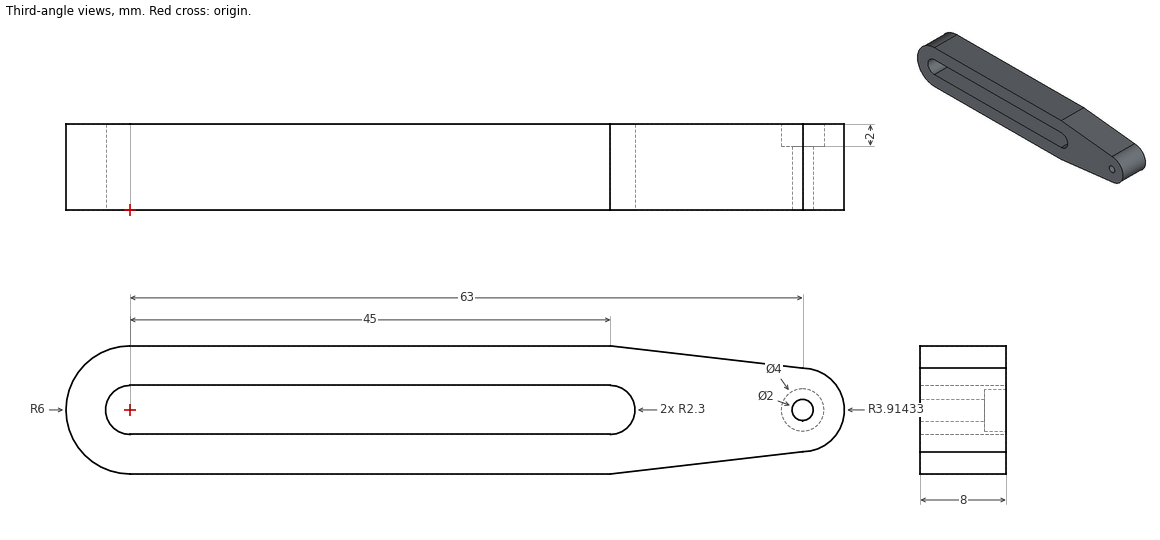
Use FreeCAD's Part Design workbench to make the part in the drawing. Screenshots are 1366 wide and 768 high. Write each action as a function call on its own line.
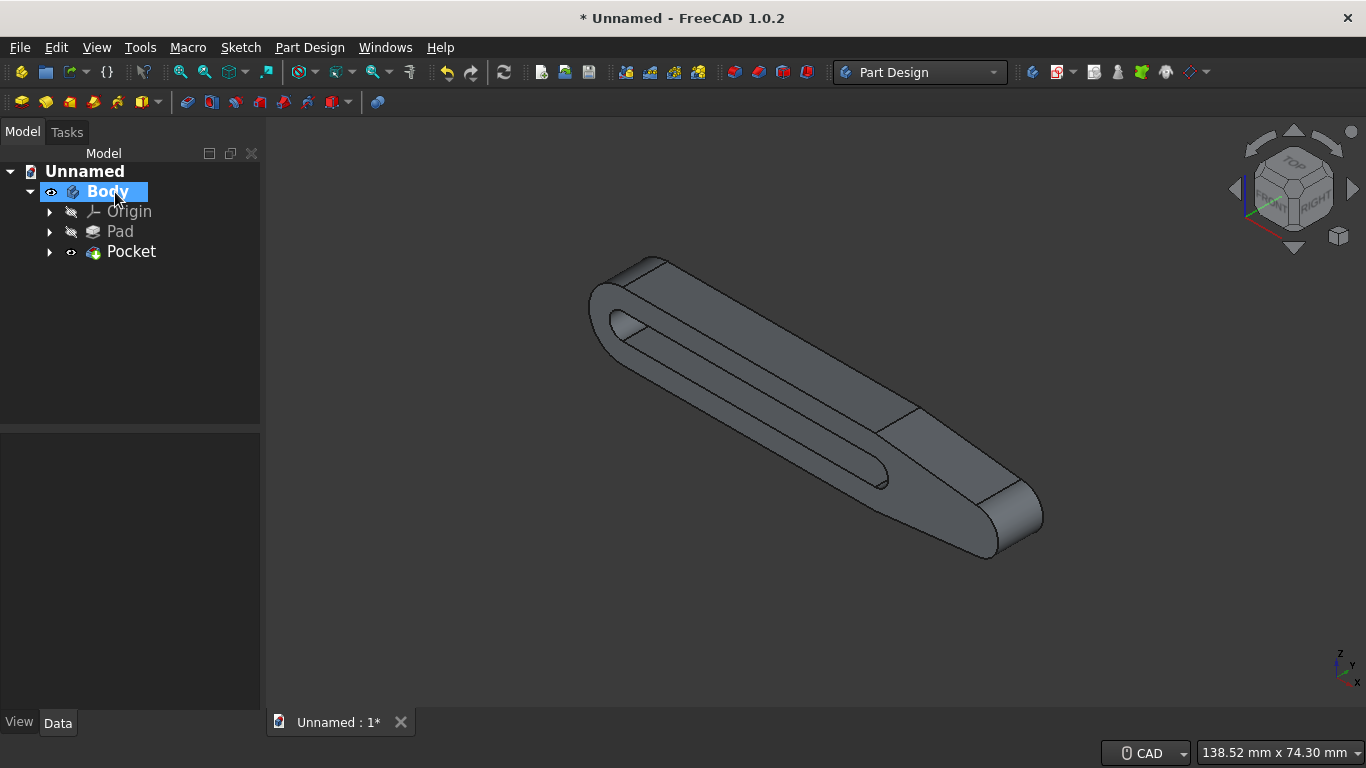
click(969, 525)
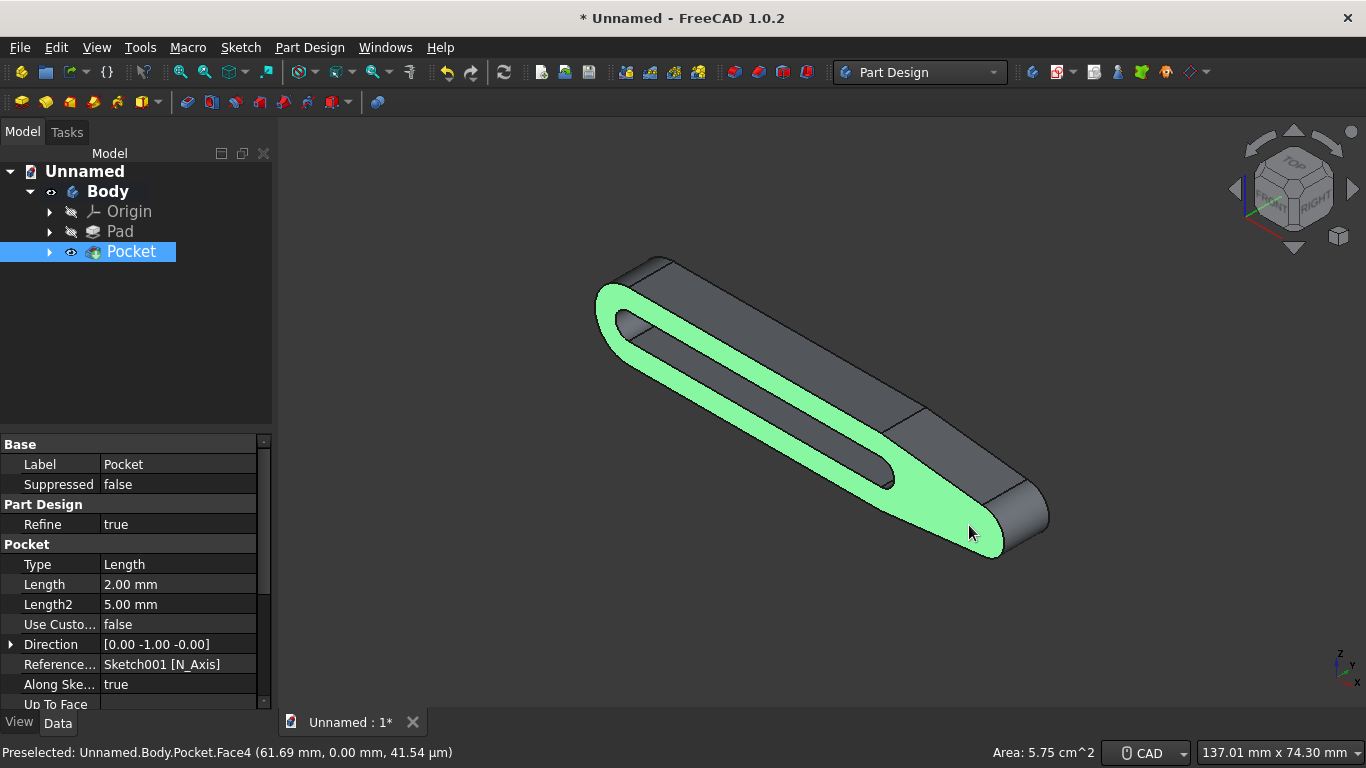
click(1058, 72)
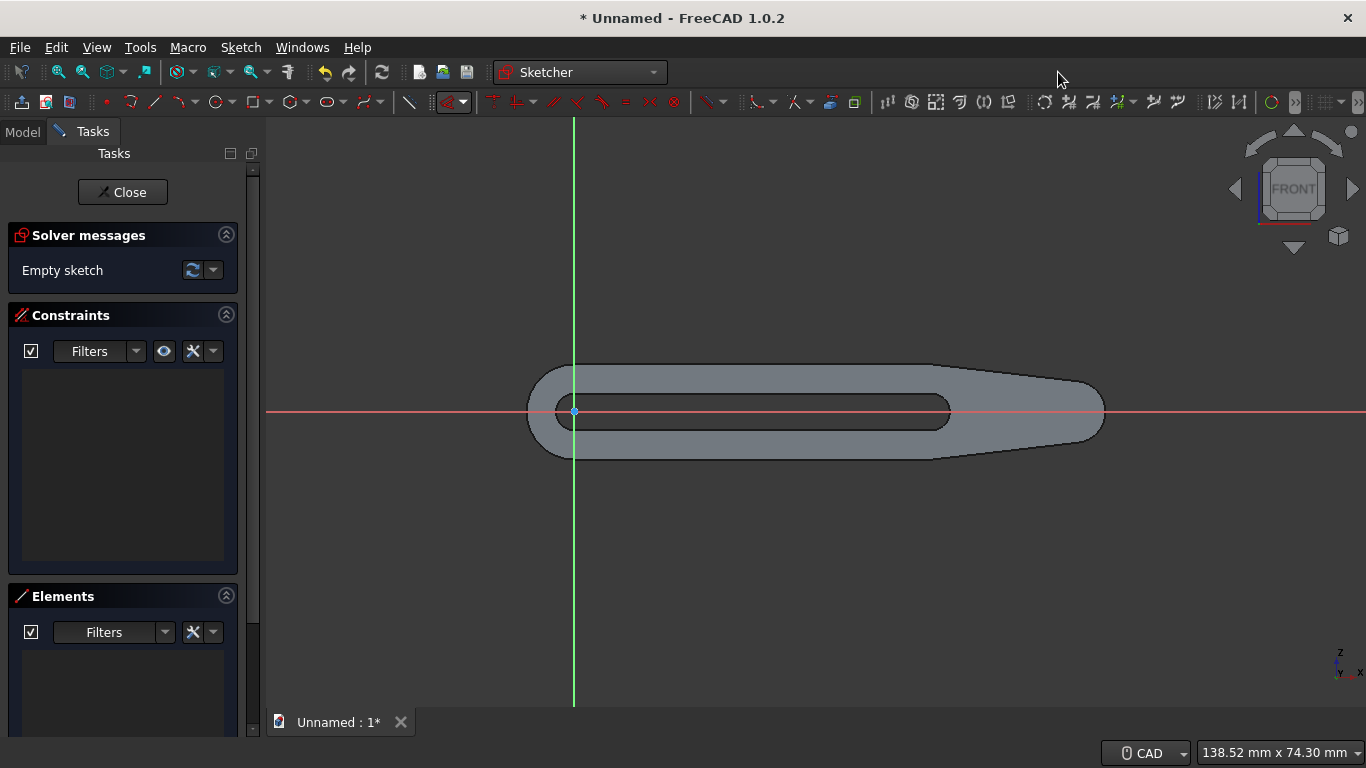
scroll(1092, 412, up, 15)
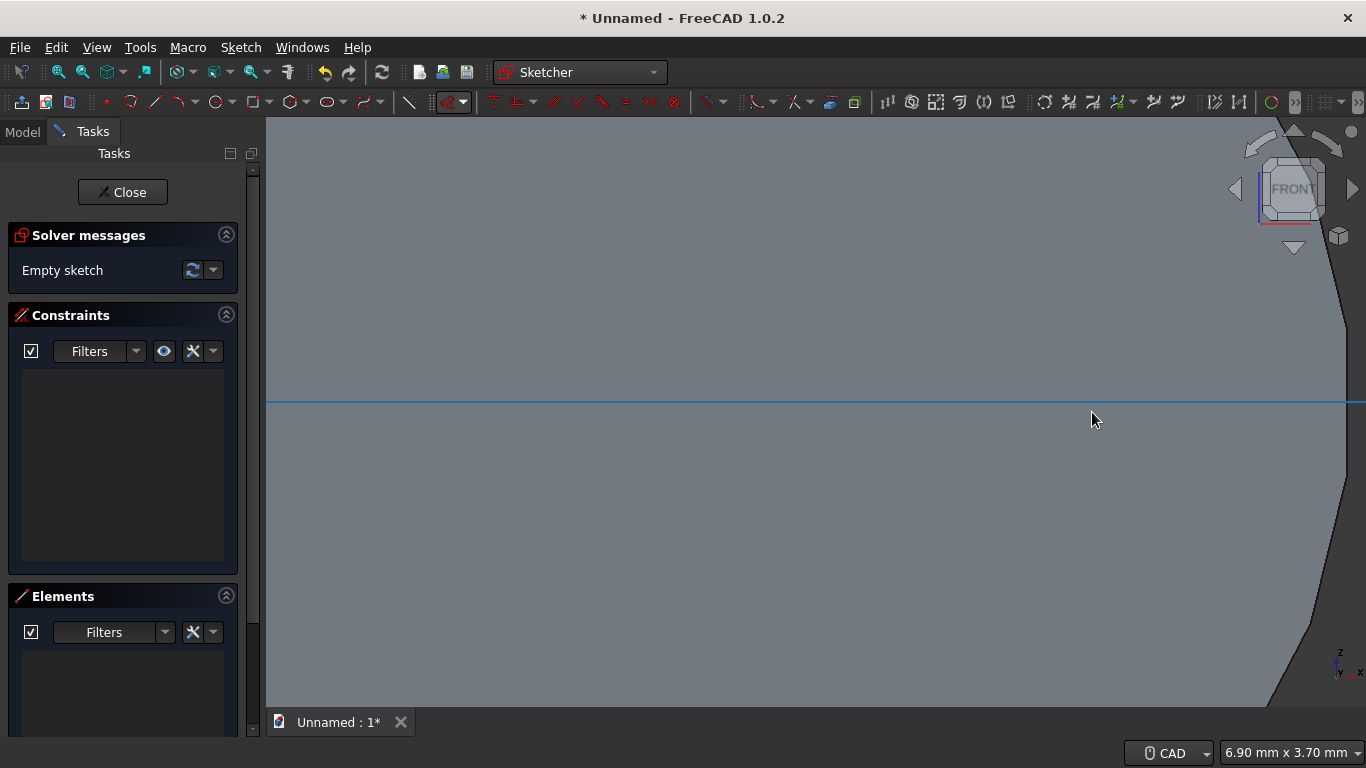
click(216, 102)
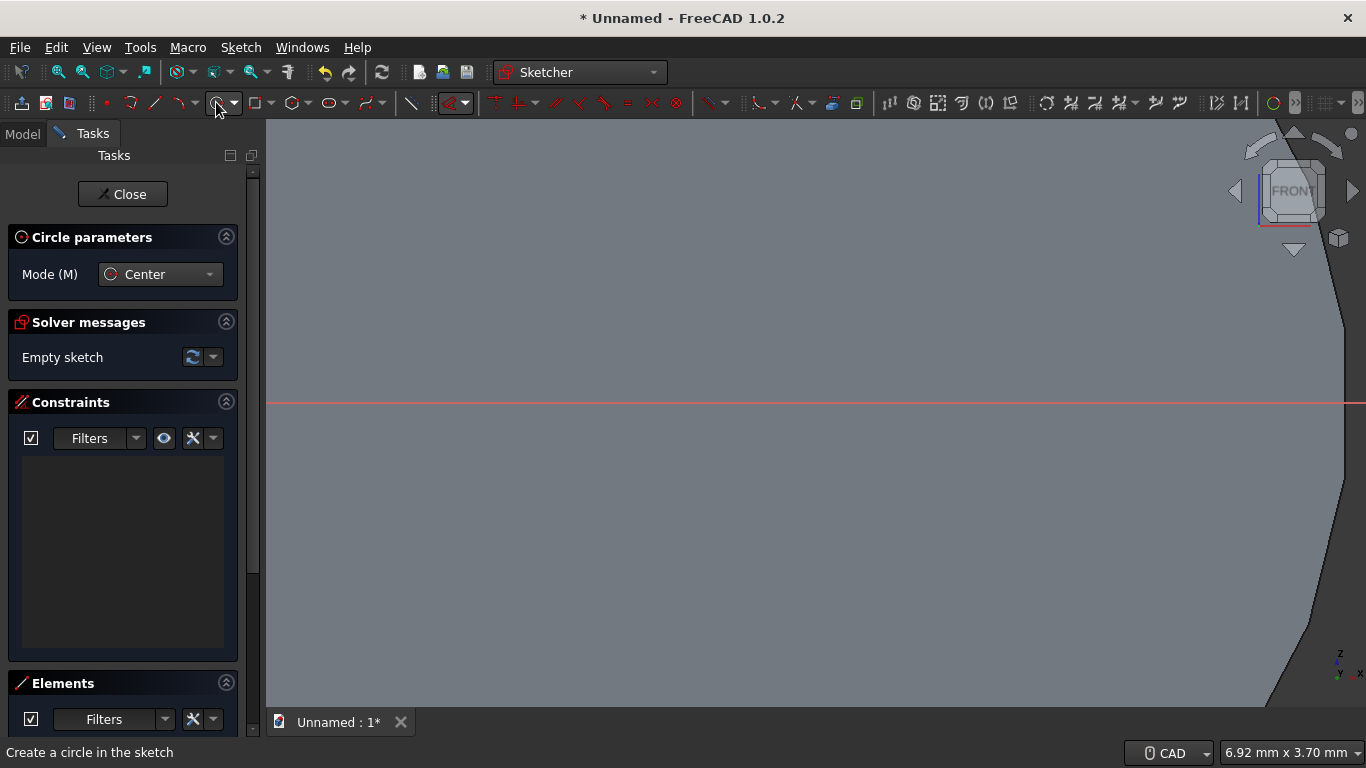
click(727, 403)
move(840, 291)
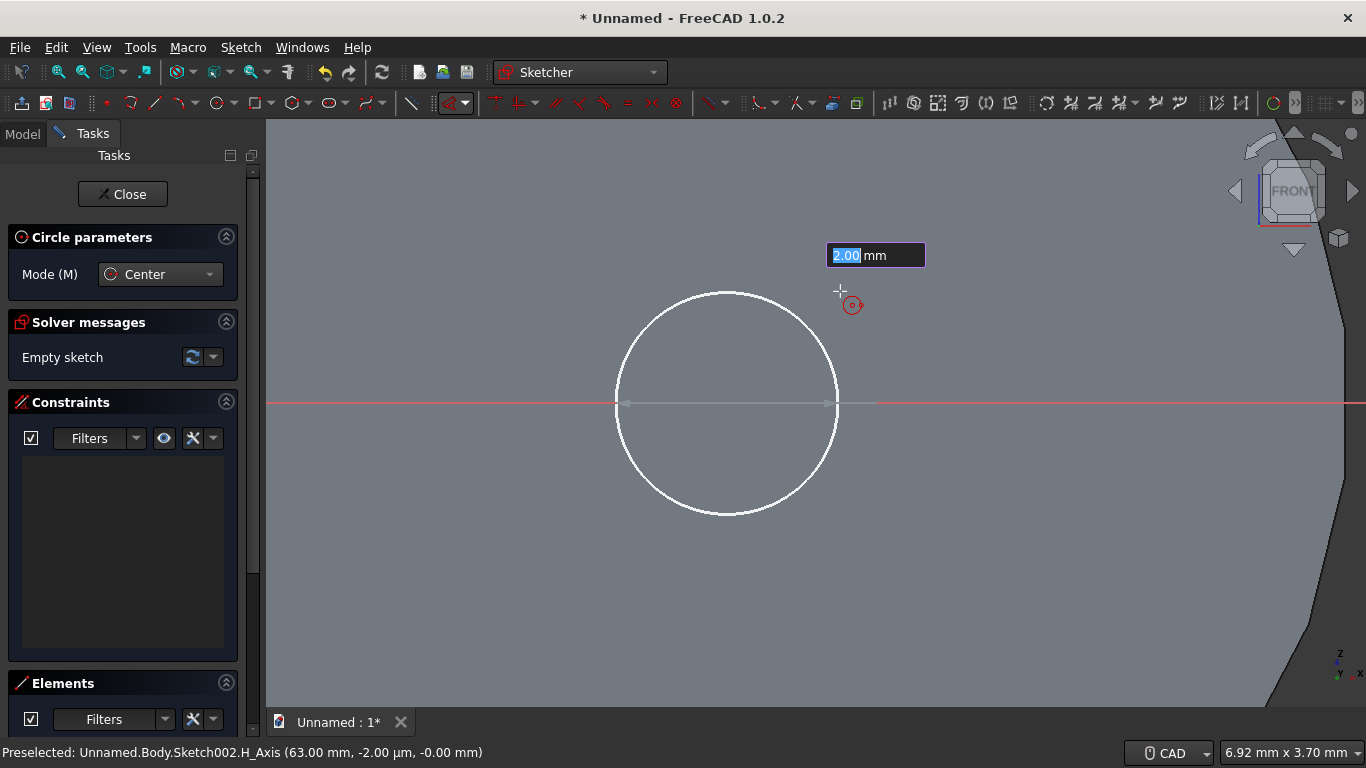
text(2)
key(Return)
key(Escape)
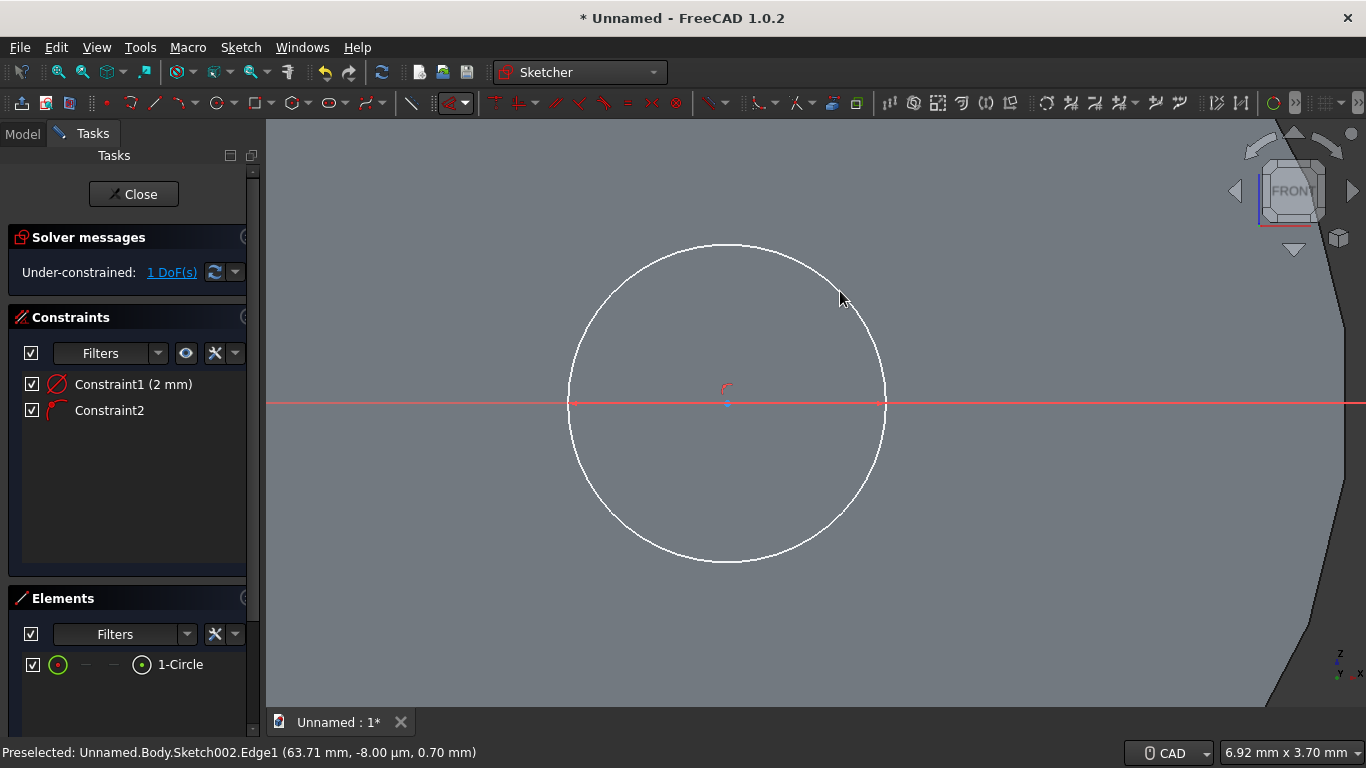
click(727, 403)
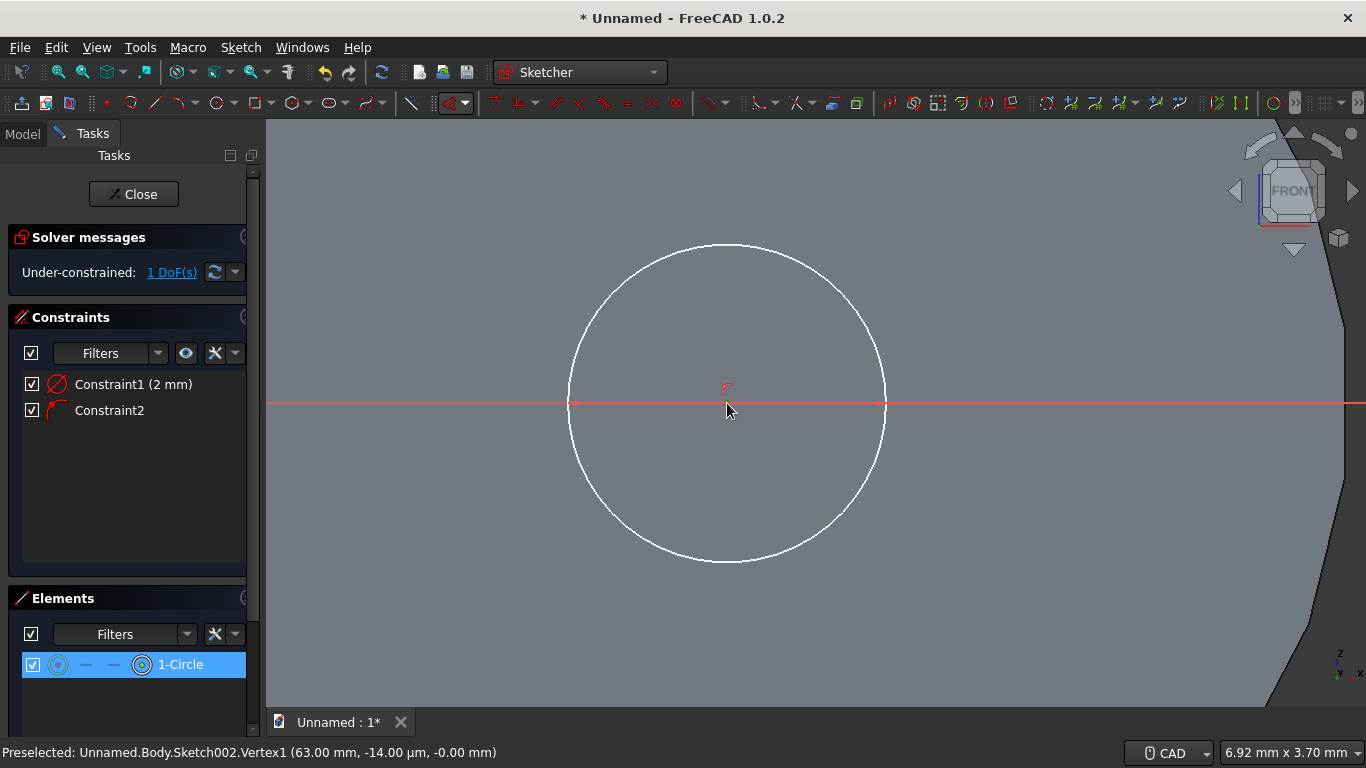
key(l)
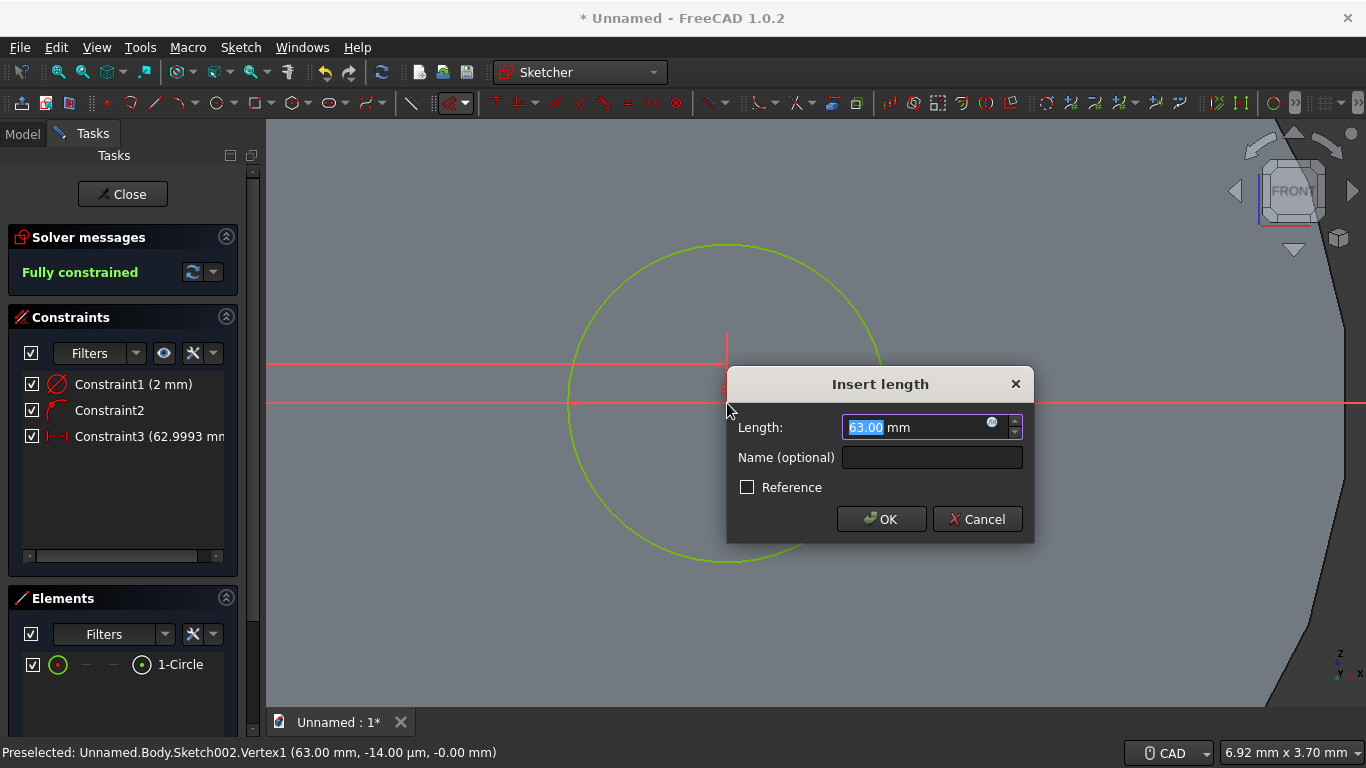
text(63)
key(Return)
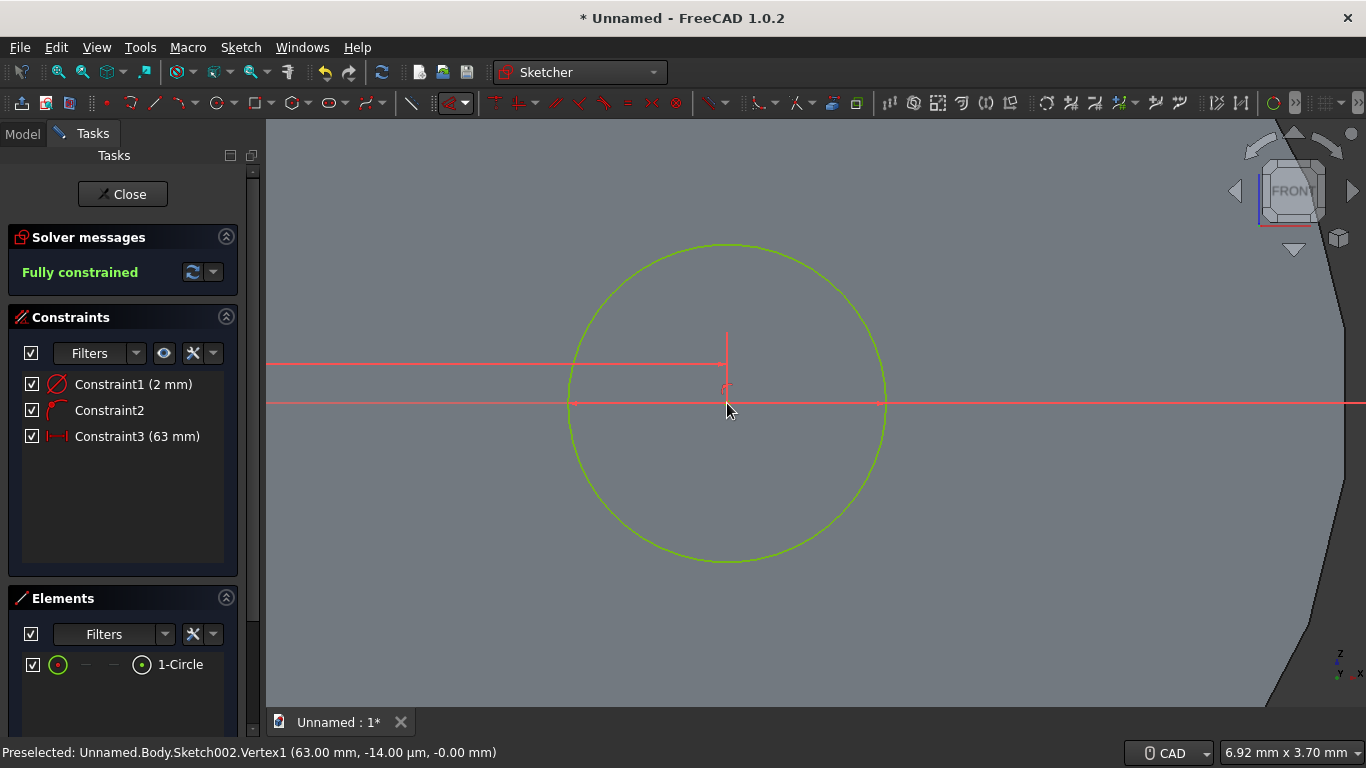
click(123, 194)